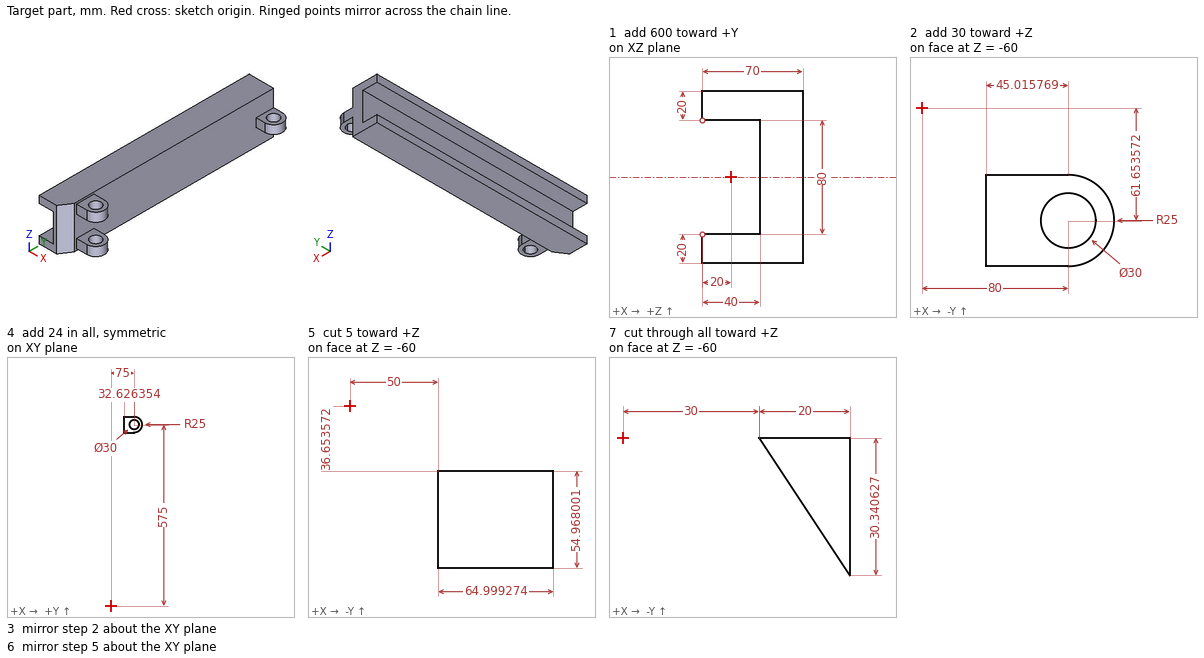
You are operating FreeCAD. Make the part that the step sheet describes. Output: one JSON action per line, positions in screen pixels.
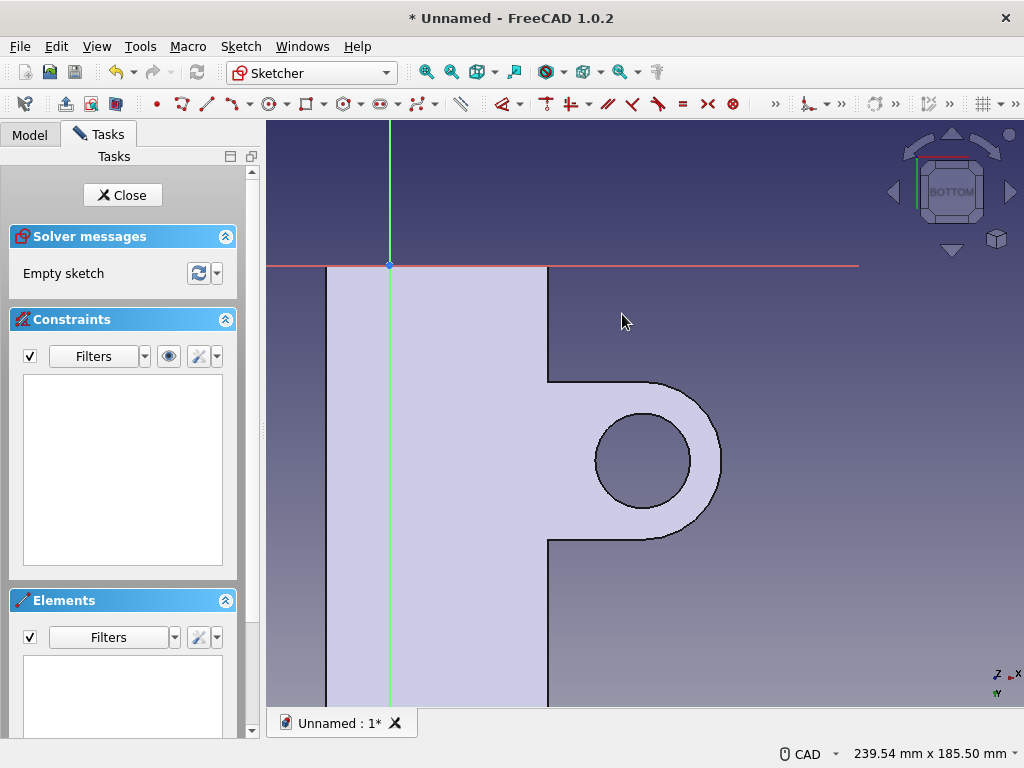
{"action": "left_click", "coordinate": [306, 104]}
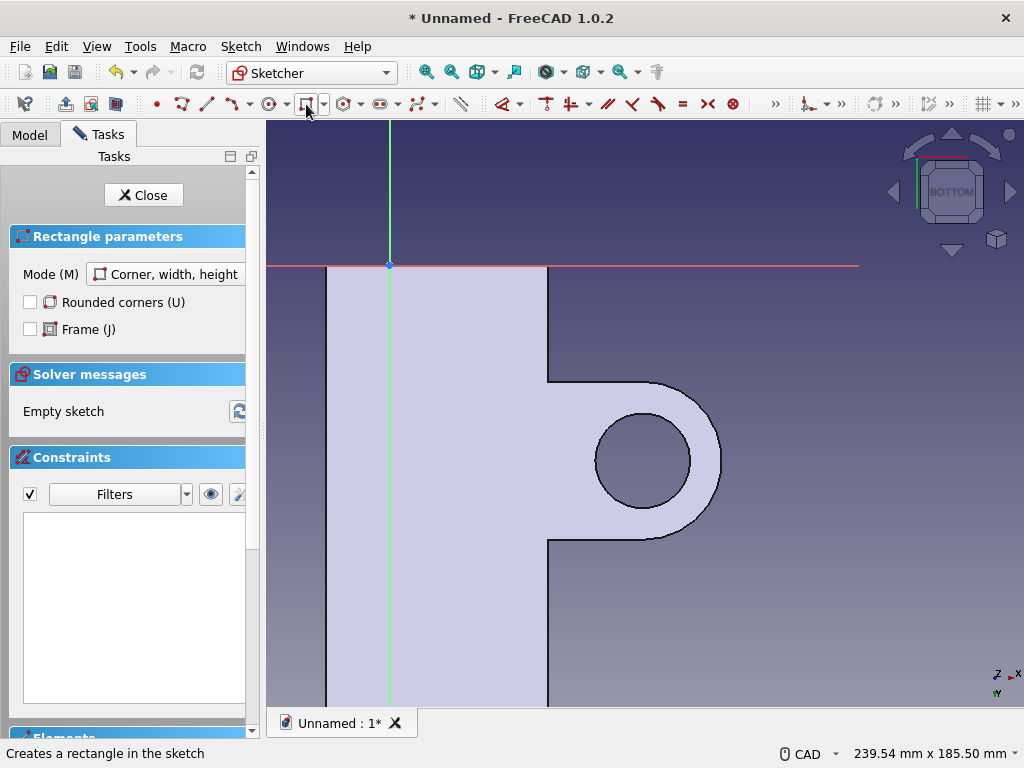
{"action": "left_click", "coordinate": [548, 382]}
{"action": "mouse_move", "coordinate": [754, 556]}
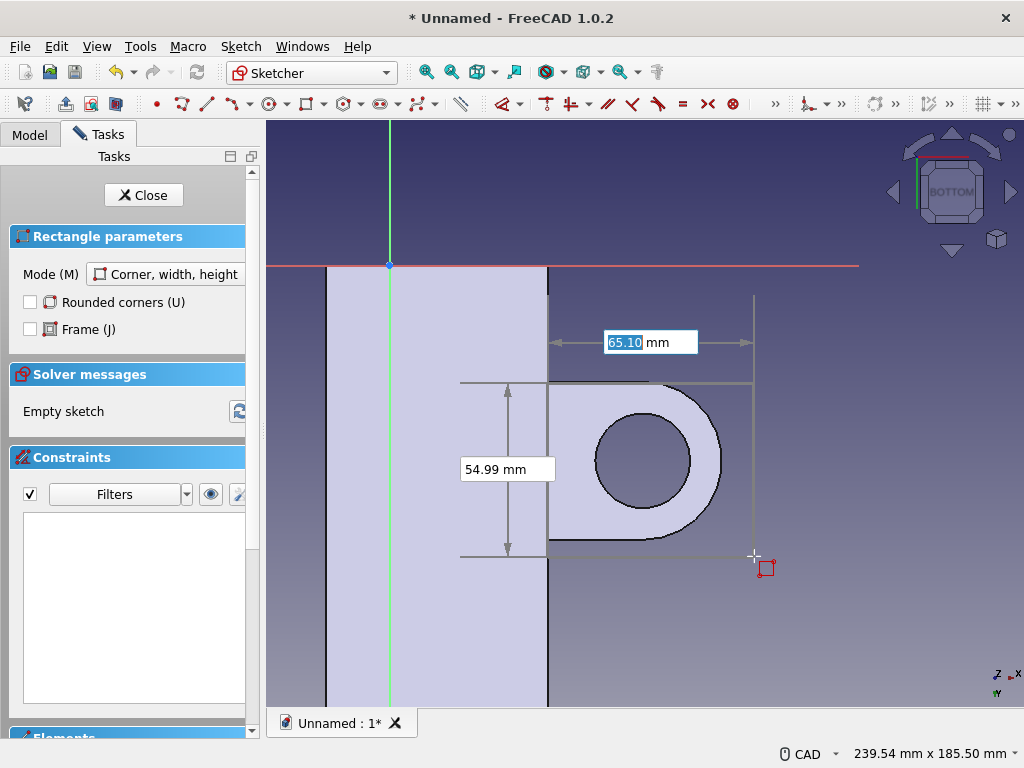
{"action": "type", "text": "64.999274"}
{"action": "key", "text": "Tab"}
{"action": "type", "text": "54.968001"}
{"action": "key", "text": "Return"}
{"action": "key", "text": "Escape"}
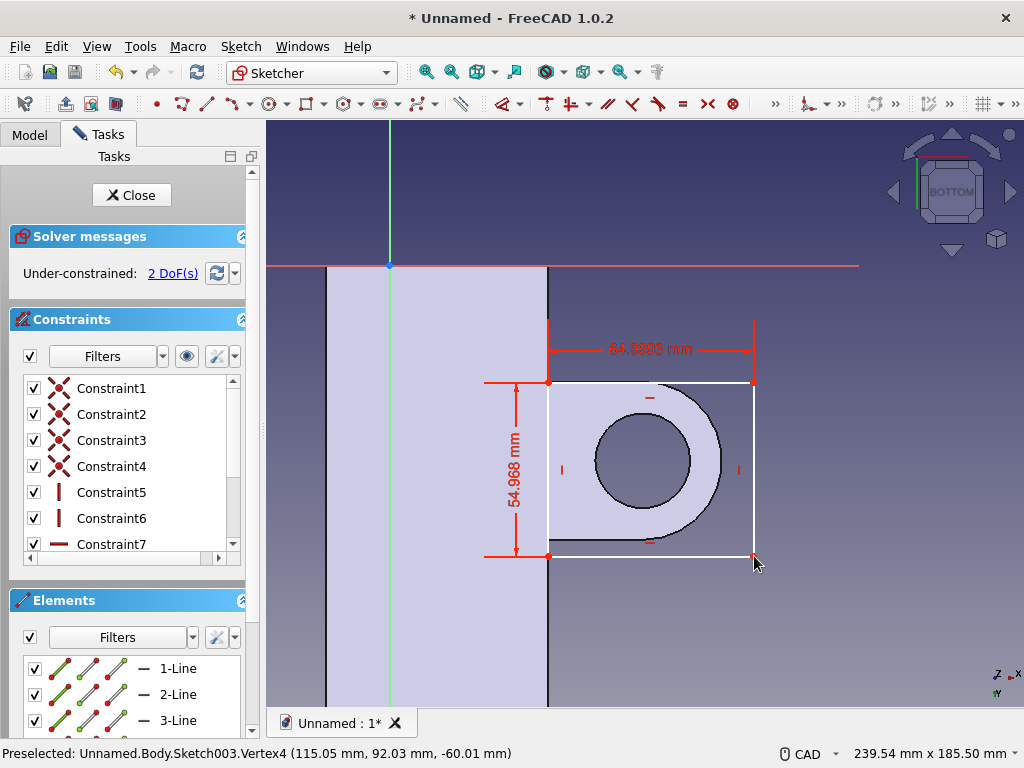
{"action": "left_click", "coordinate": [502, 104]}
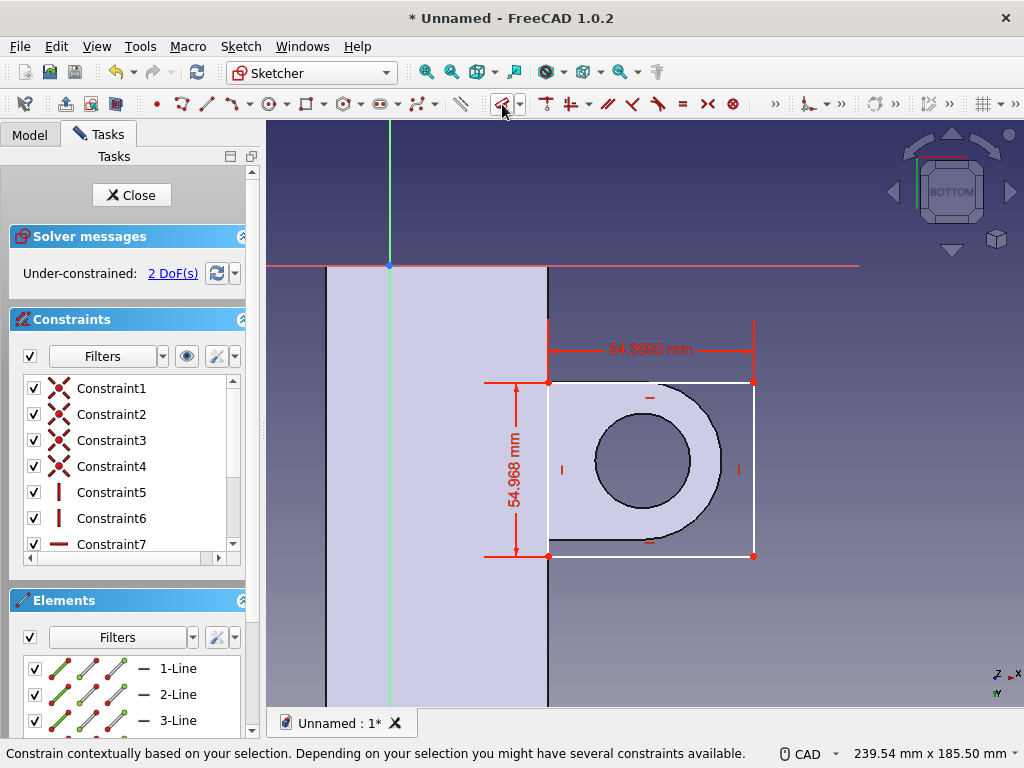
{"action": "left_click", "coordinate": [548, 383]}
{"action": "left_click", "coordinate": [469, 232]}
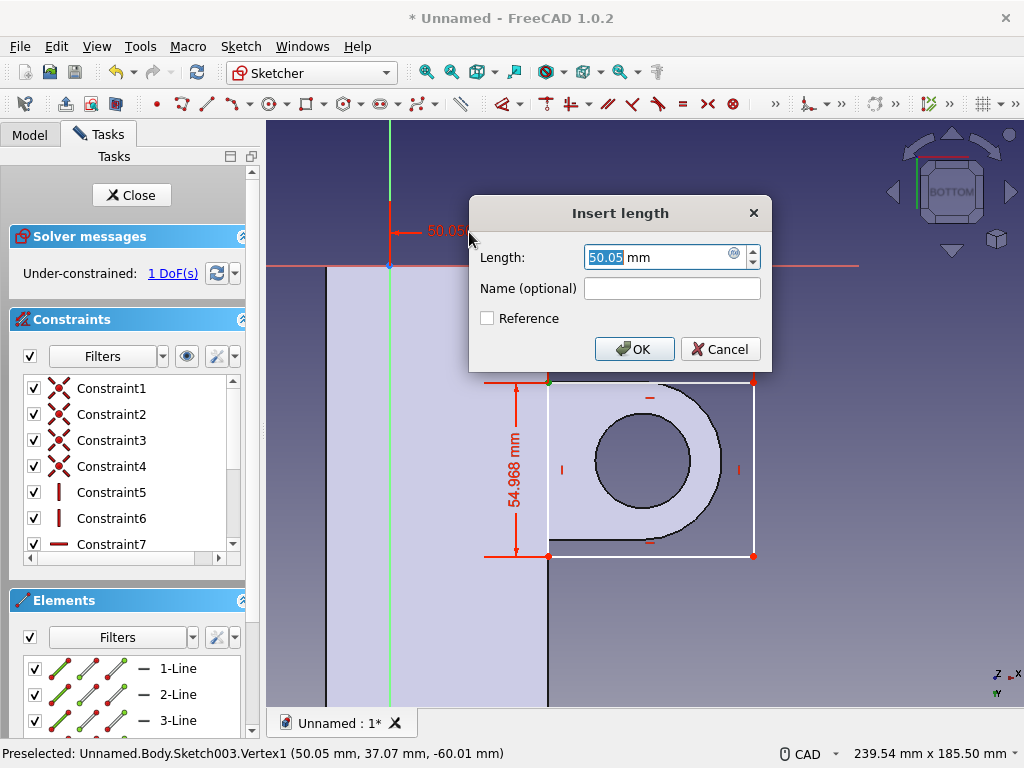
{"action": "type", "text": "50"}
{"action": "key", "text": "Return"}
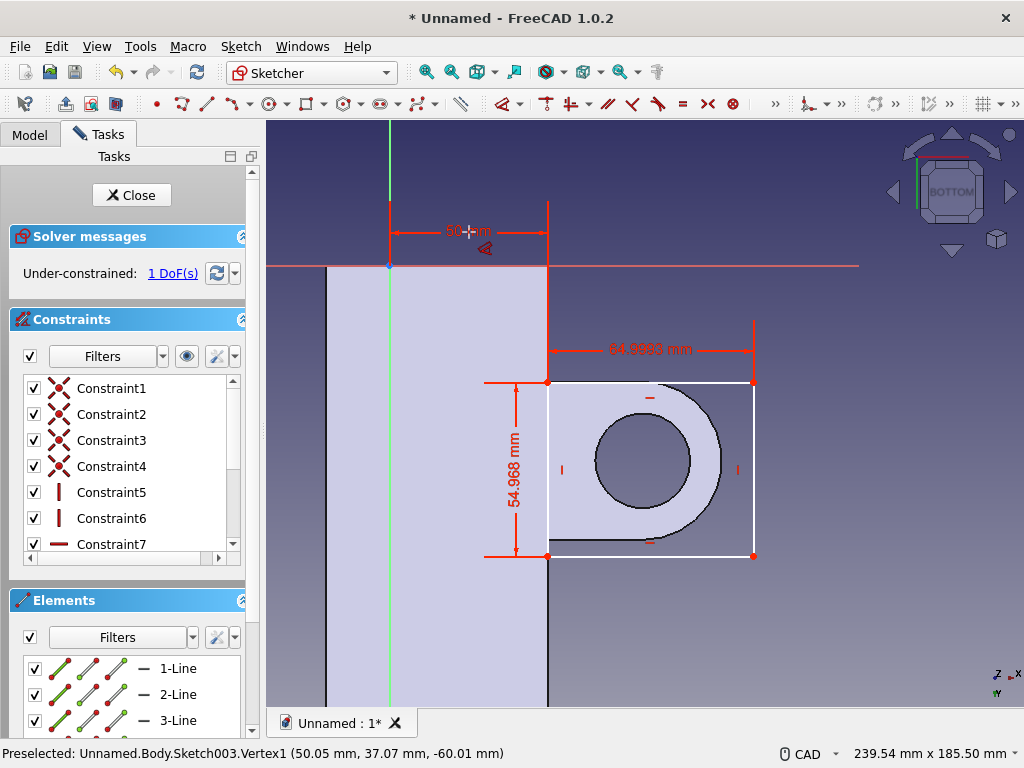
{"action": "left_click", "coordinate": [548, 383]}
{"action": "left_click", "coordinate": [356, 324]}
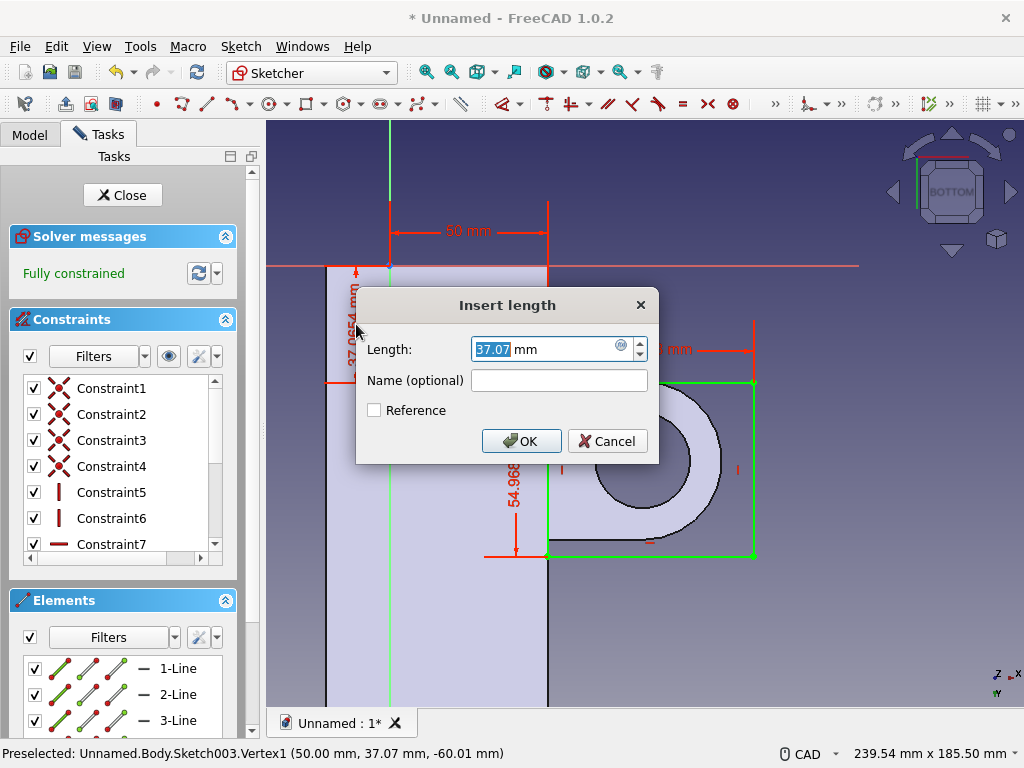
{"action": "type", "text": "36.653572"}
{"action": "key", "text": "Return"}
{"action": "key", "text": "Escape"}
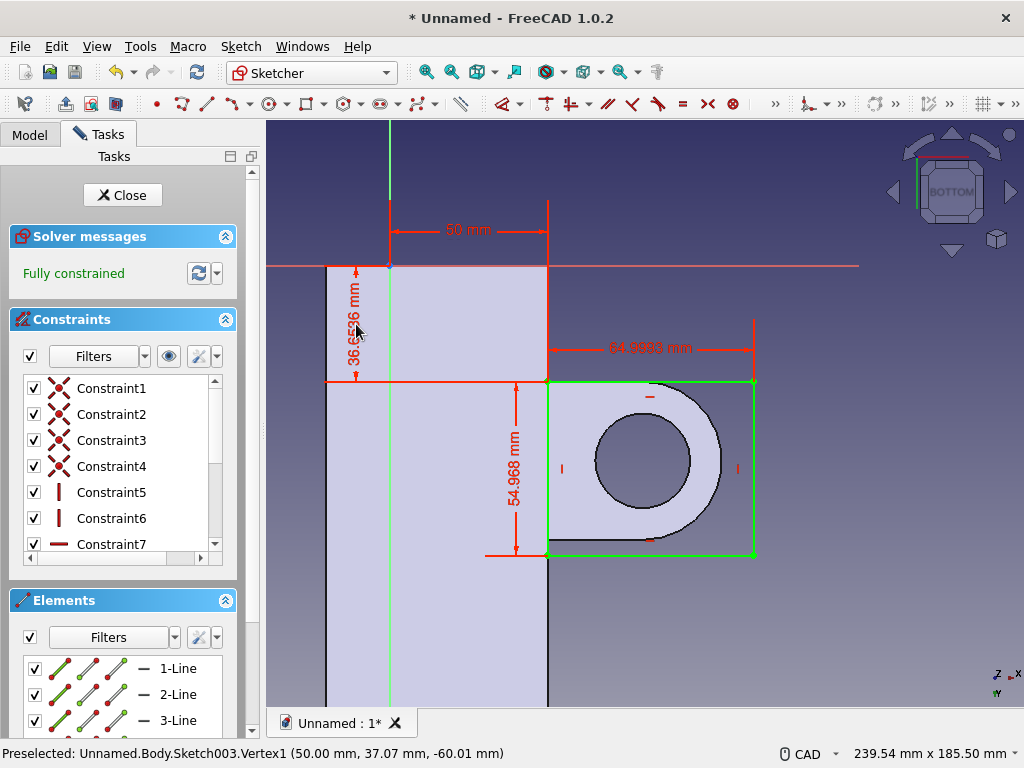
{"action": "left_click", "coordinate": [123, 195]}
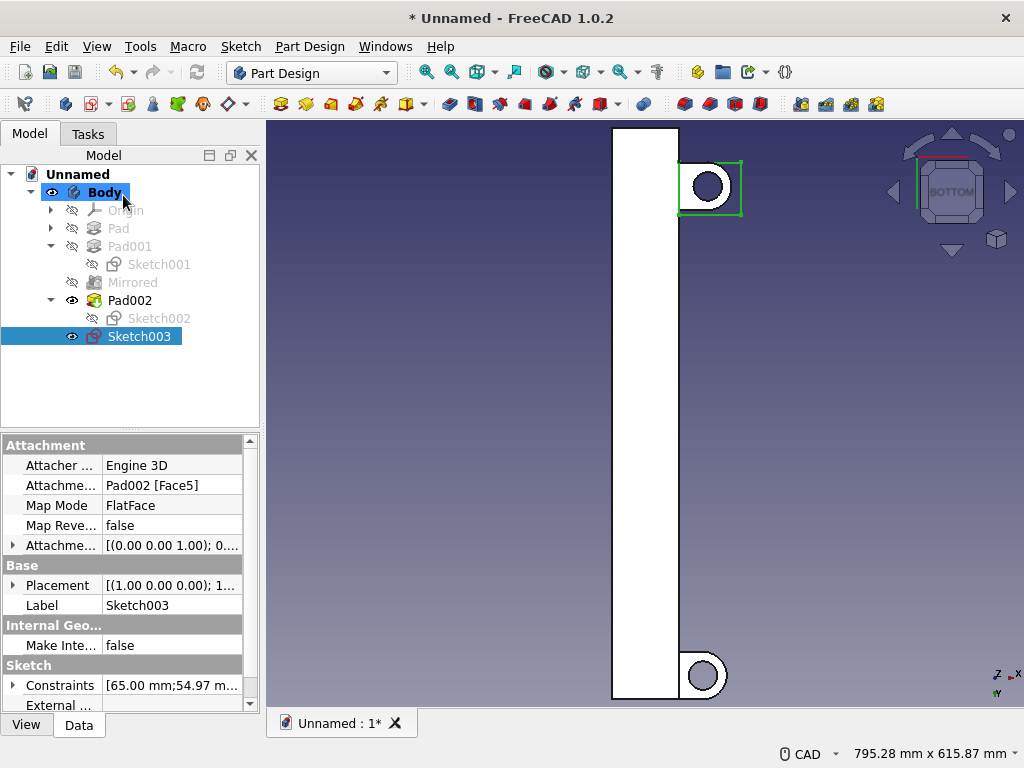
{"action": "left_click", "coordinate": [450, 104]}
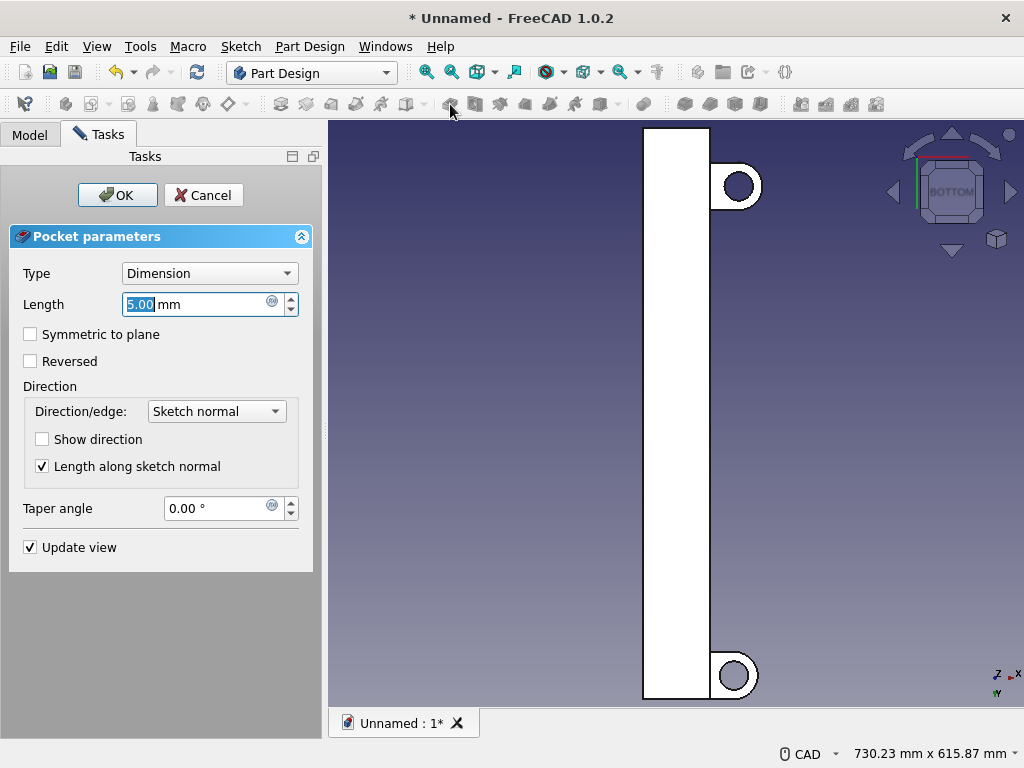
{"action": "type", "text": "5"}
{"action": "key", "text": "Tab"}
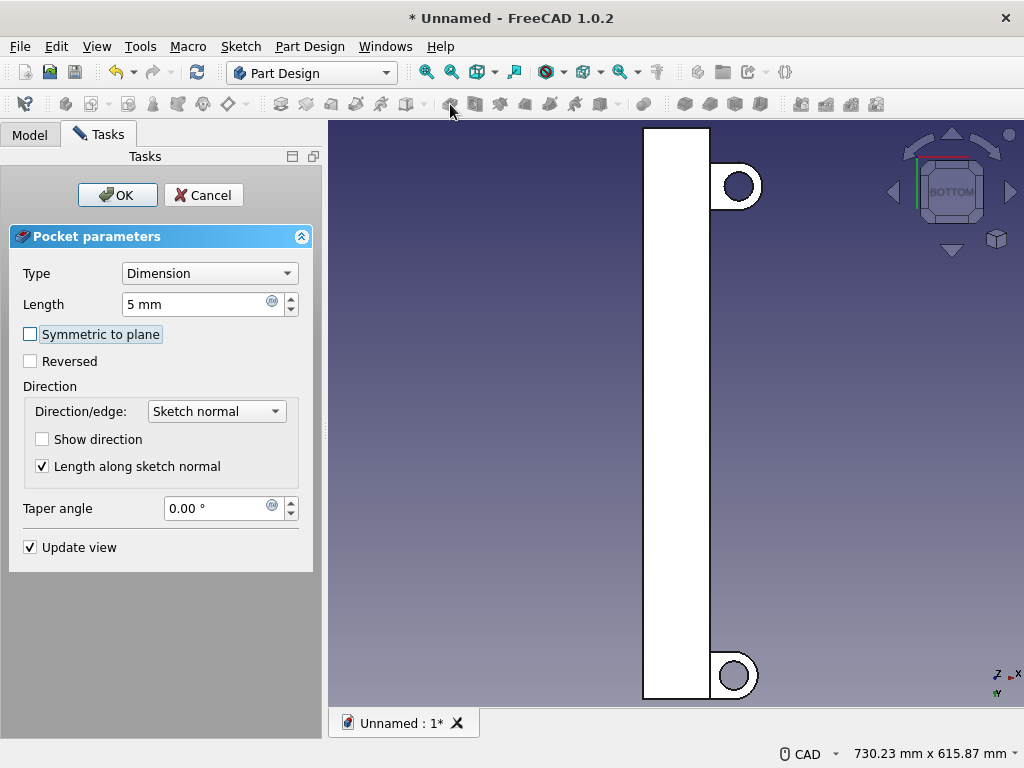
{"action": "left_click", "coordinate": [118, 195]}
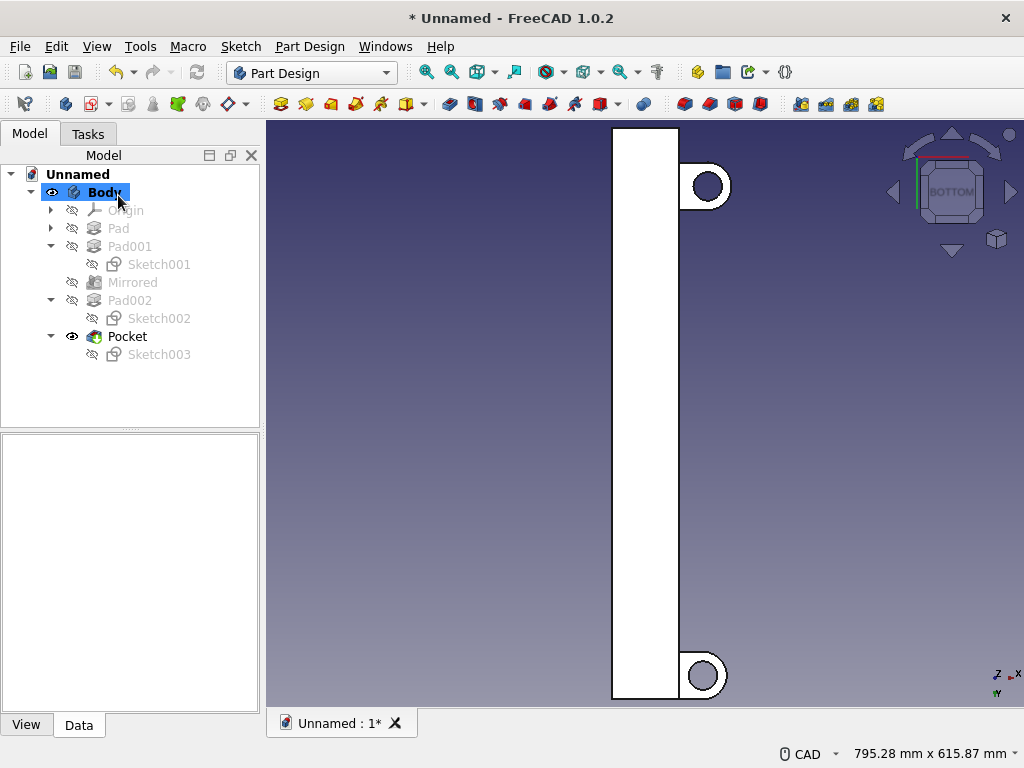
{"action": "left_click", "coordinate": [117, 336]}